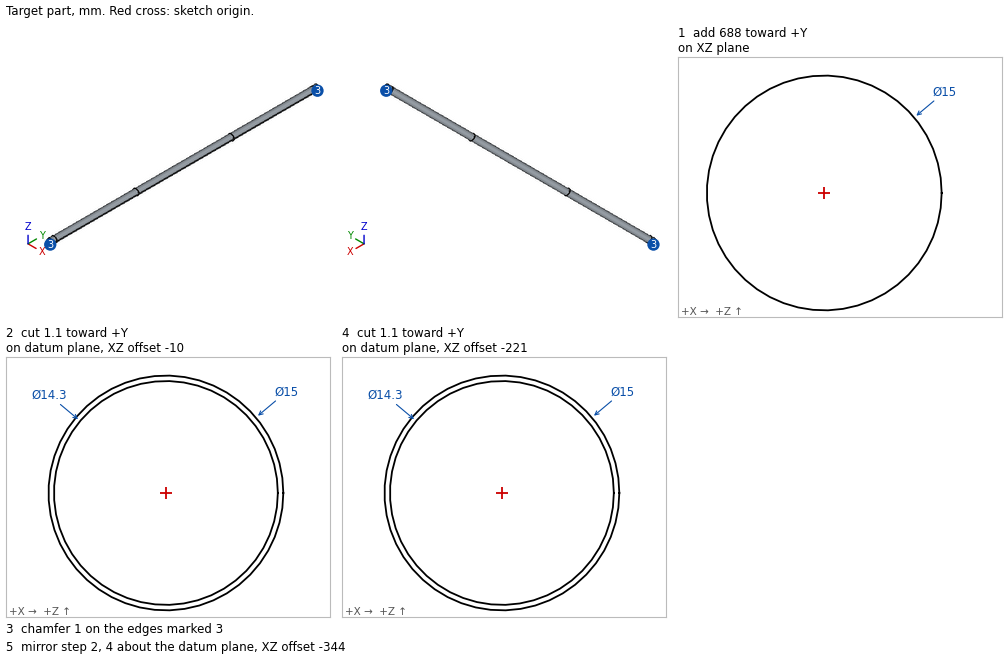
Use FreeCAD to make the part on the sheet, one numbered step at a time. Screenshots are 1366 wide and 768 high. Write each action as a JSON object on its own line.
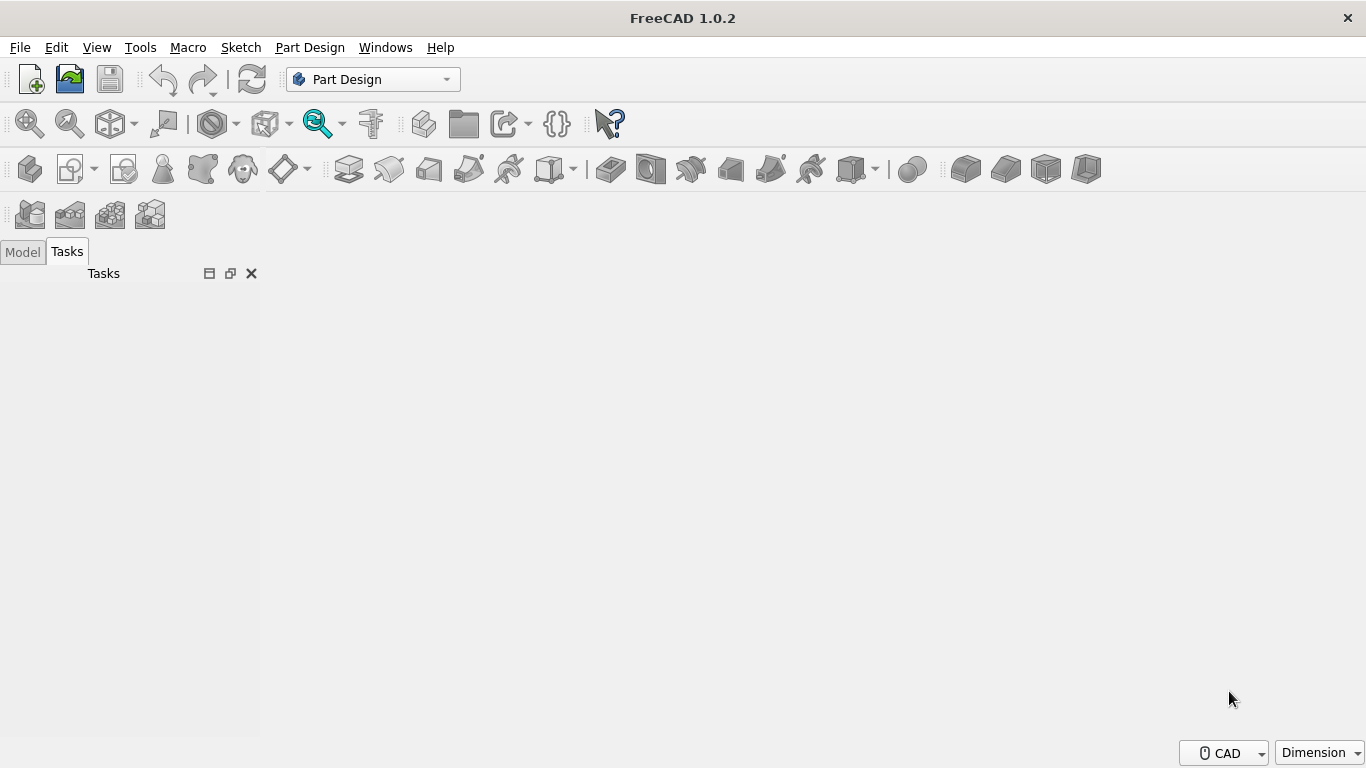
{"action": "left_click", "coordinate": [898, 80]}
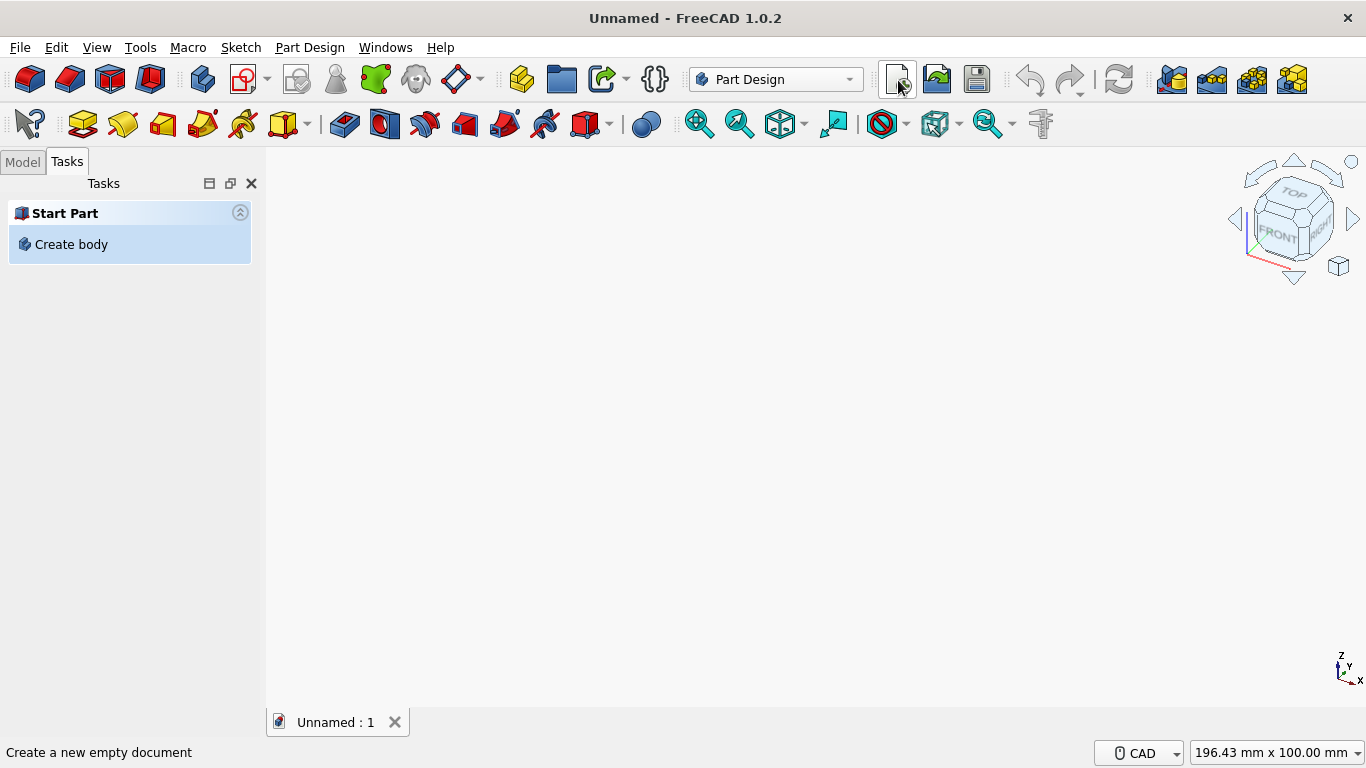
{"action": "left_click", "coordinate": [244, 80]}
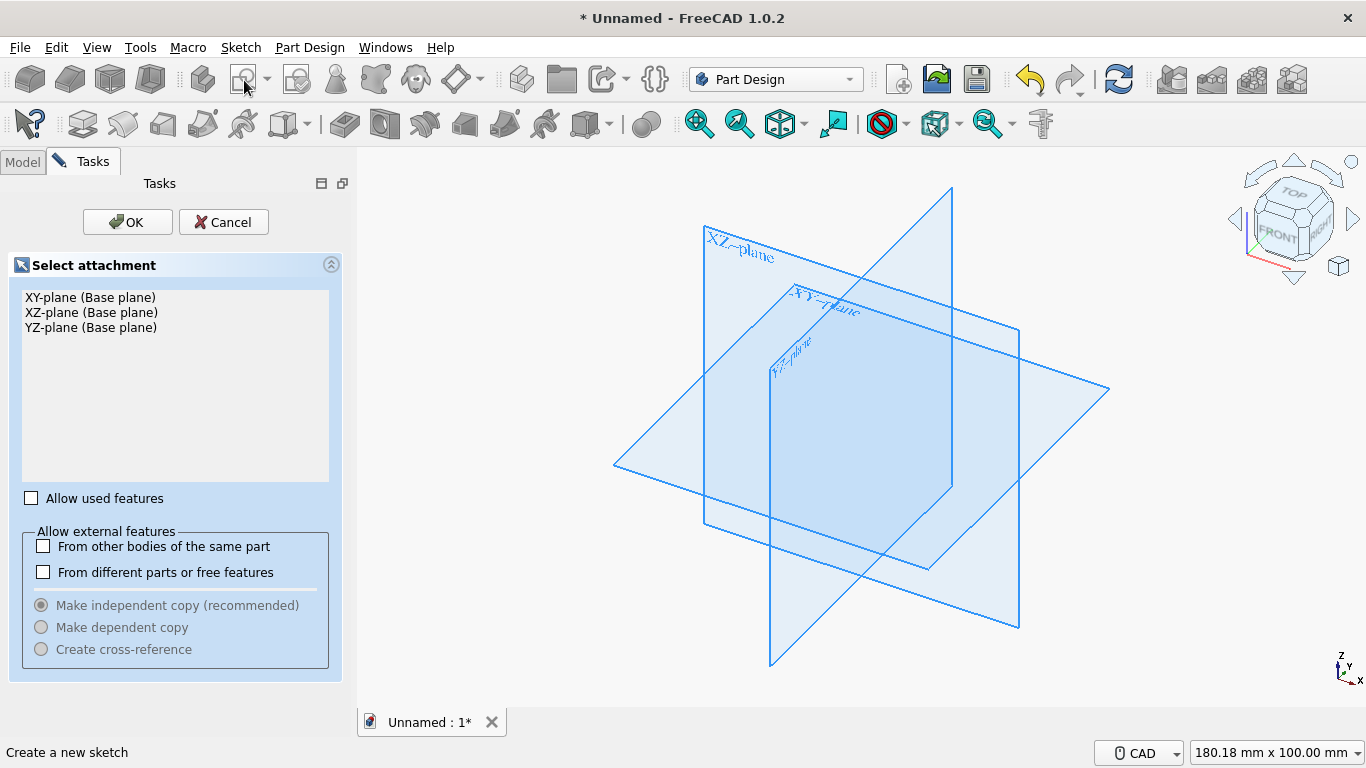
{"action": "left_click", "coordinate": [82, 312]}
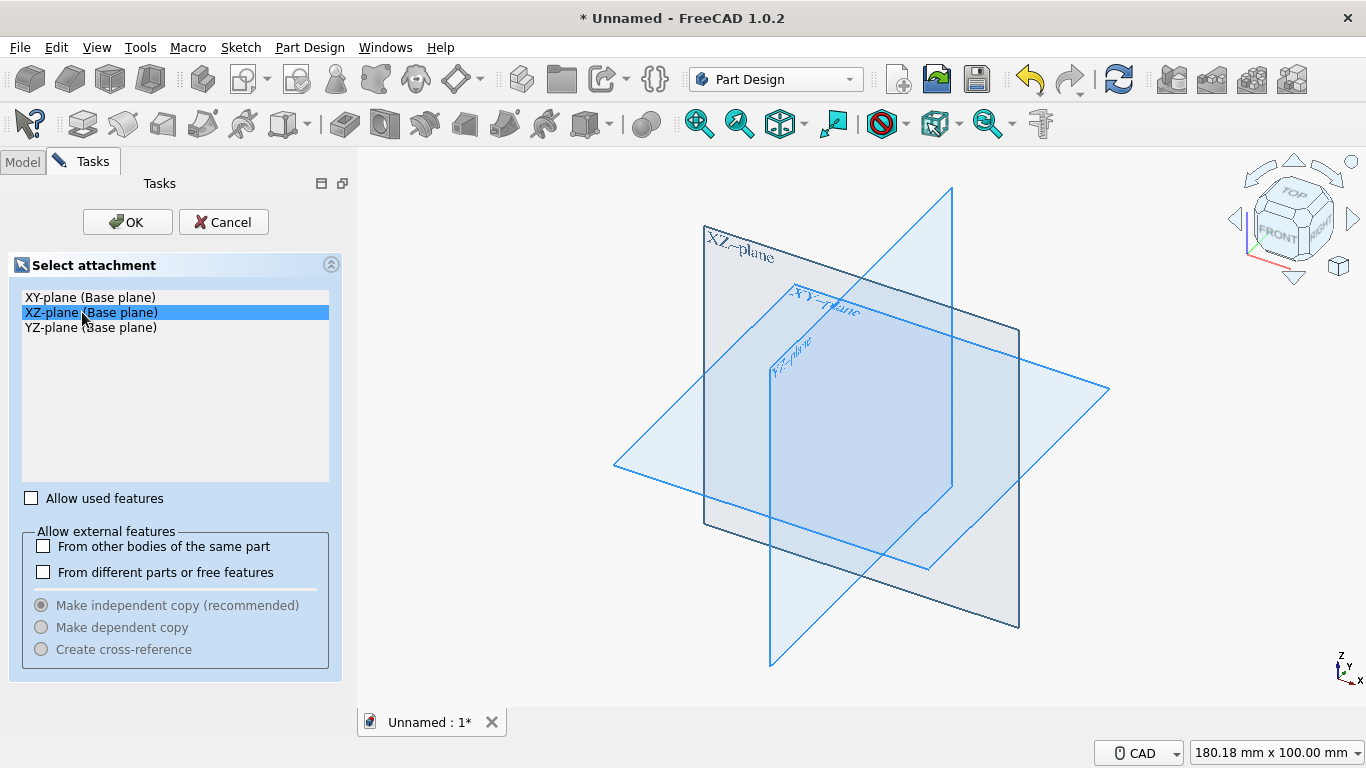
{"action": "left_click", "coordinate": [128, 222]}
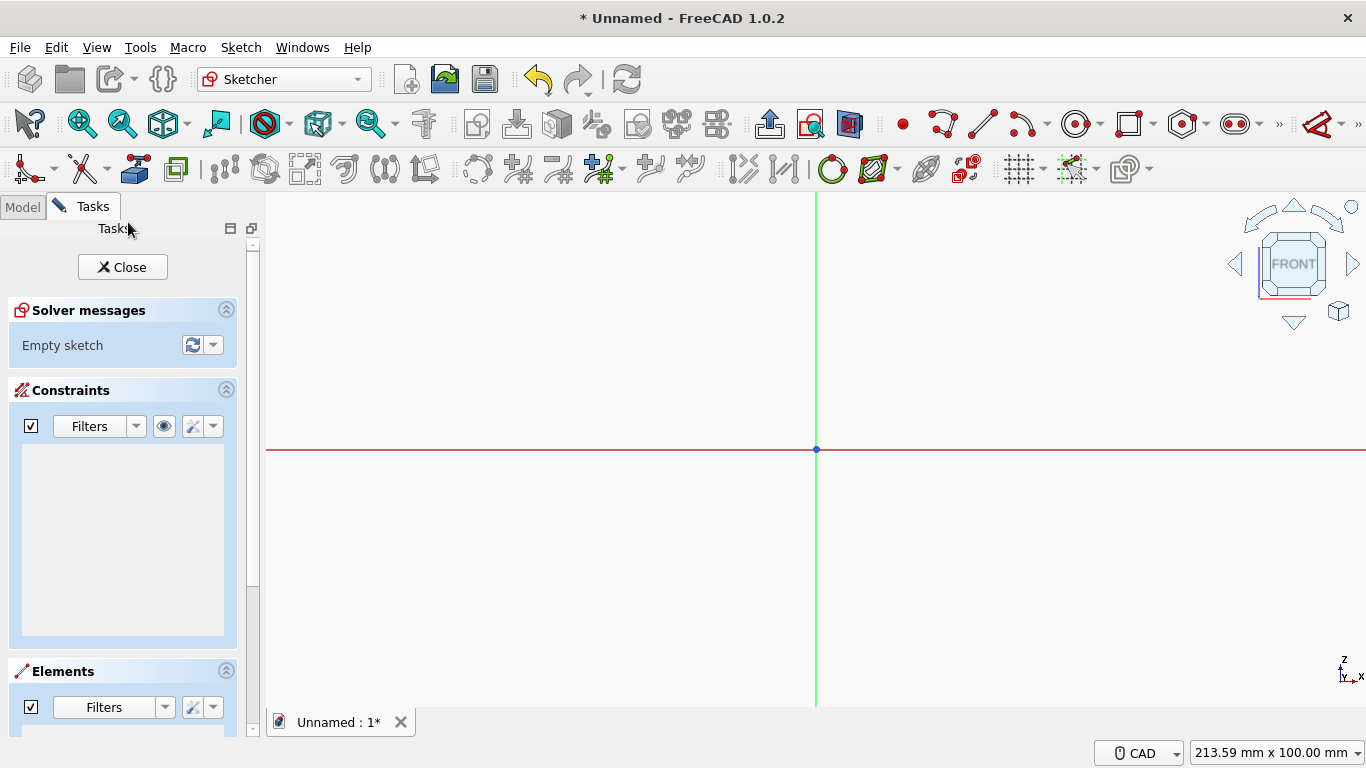
{"action": "scroll", "coordinate": [838, 449], "scroll_direction": "up", "scroll_amount": 7}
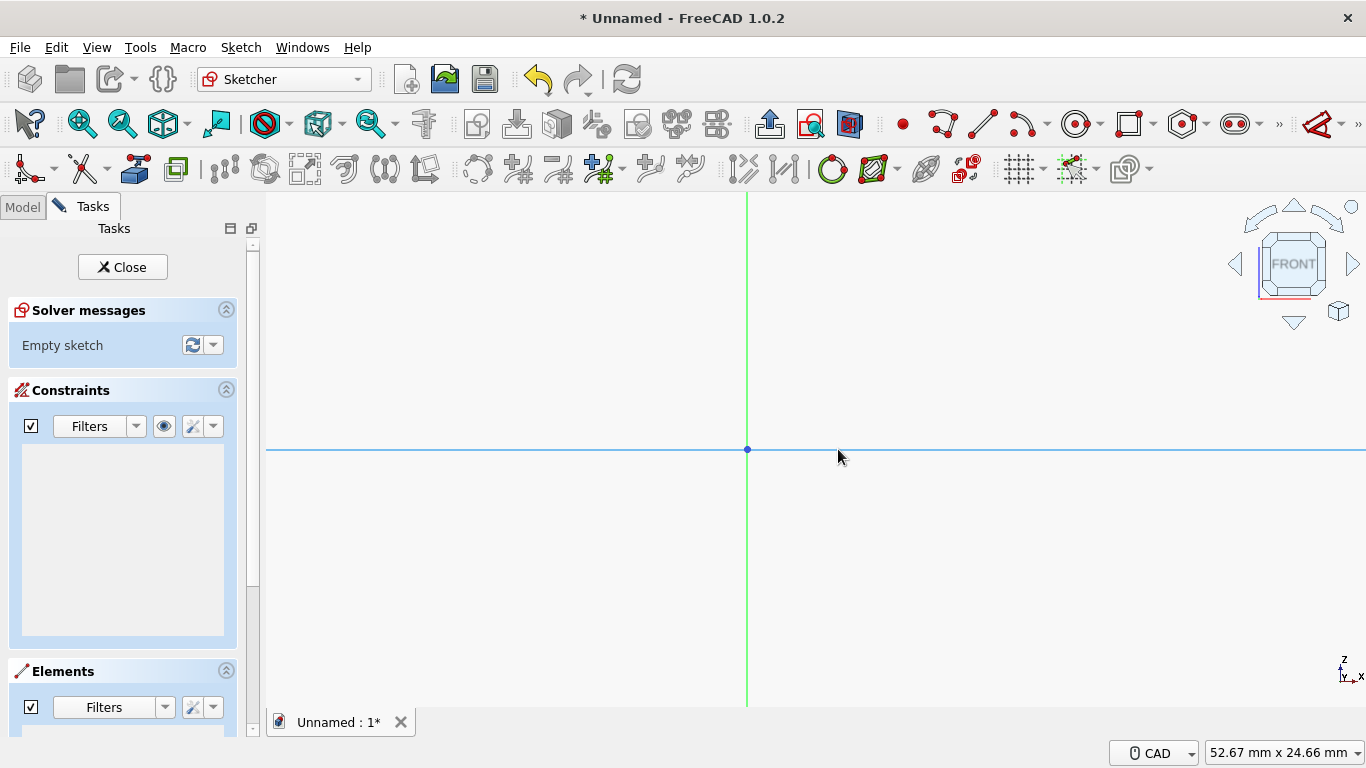
{"action": "left_click", "coordinate": [1076, 124]}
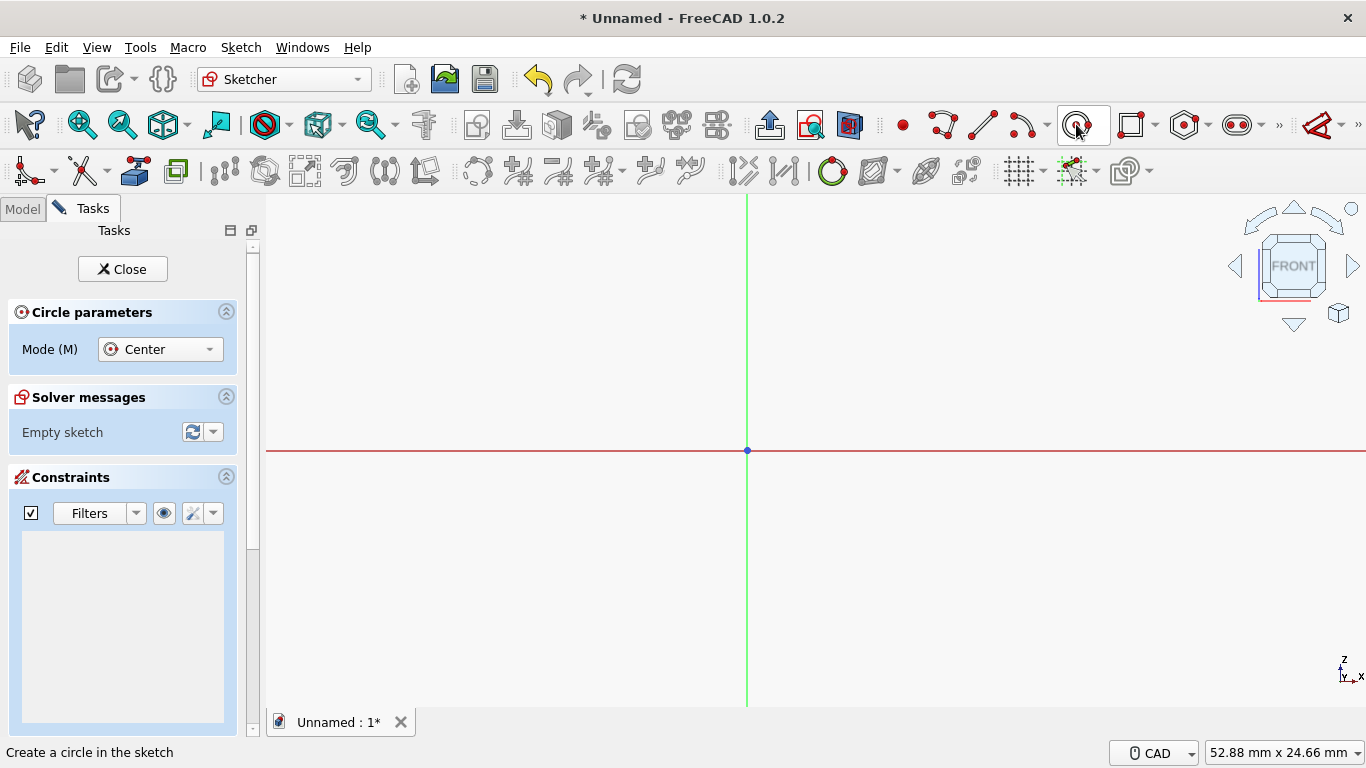
{"action": "left_click", "coordinate": [747, 450]}
{"action": "mouse_move", "coordinate": [858, 340]}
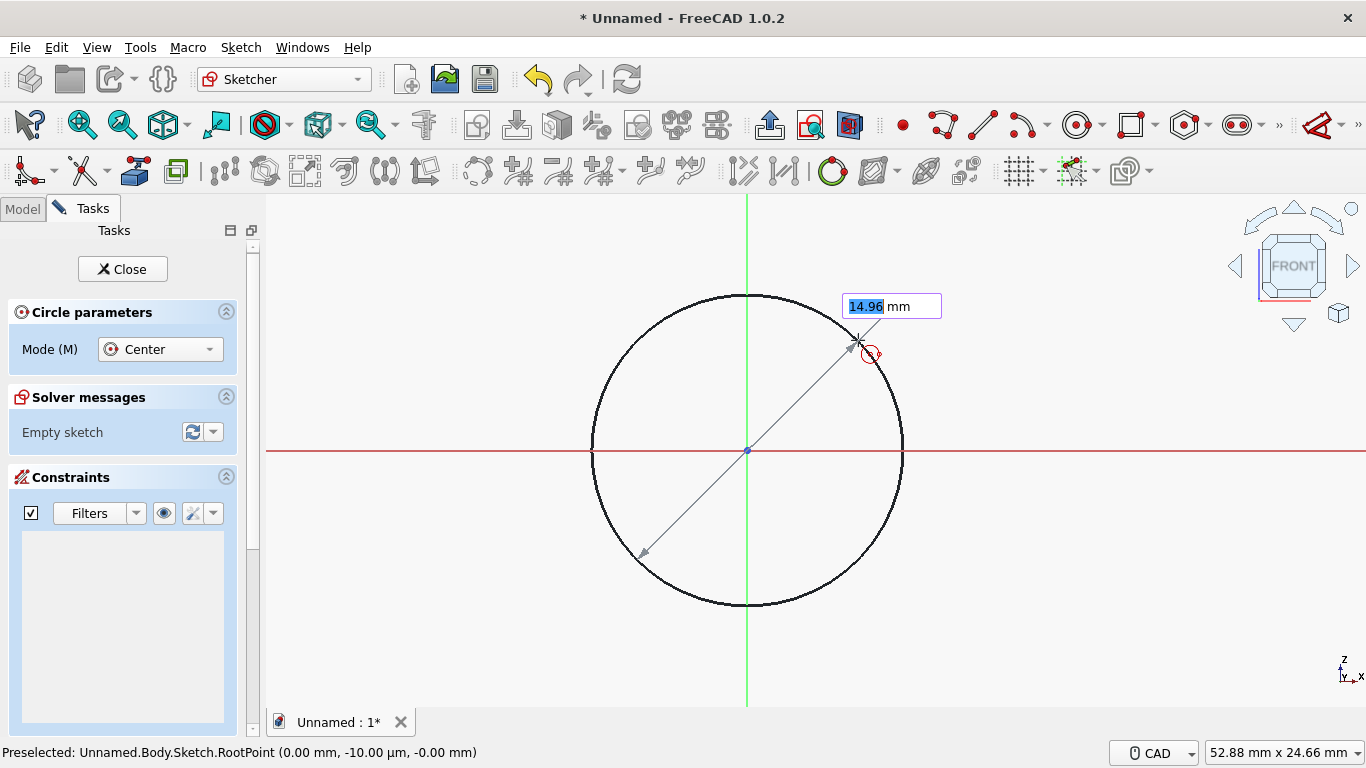
{"action": "type", "text": "15"}
{"action": "key", "text": "Return"}
{"action": "key", "text": "Escape"}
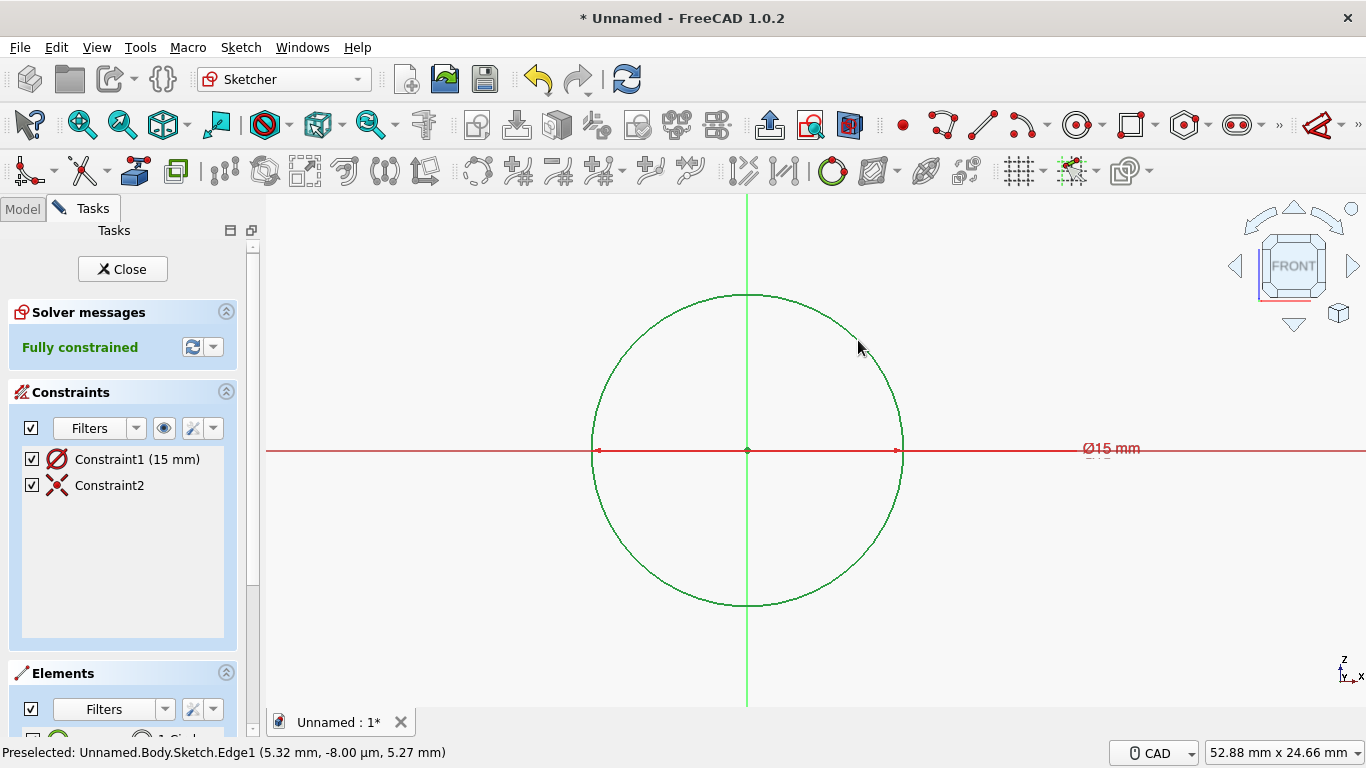
{"action": "left_click", "coordinate": [123, 269]}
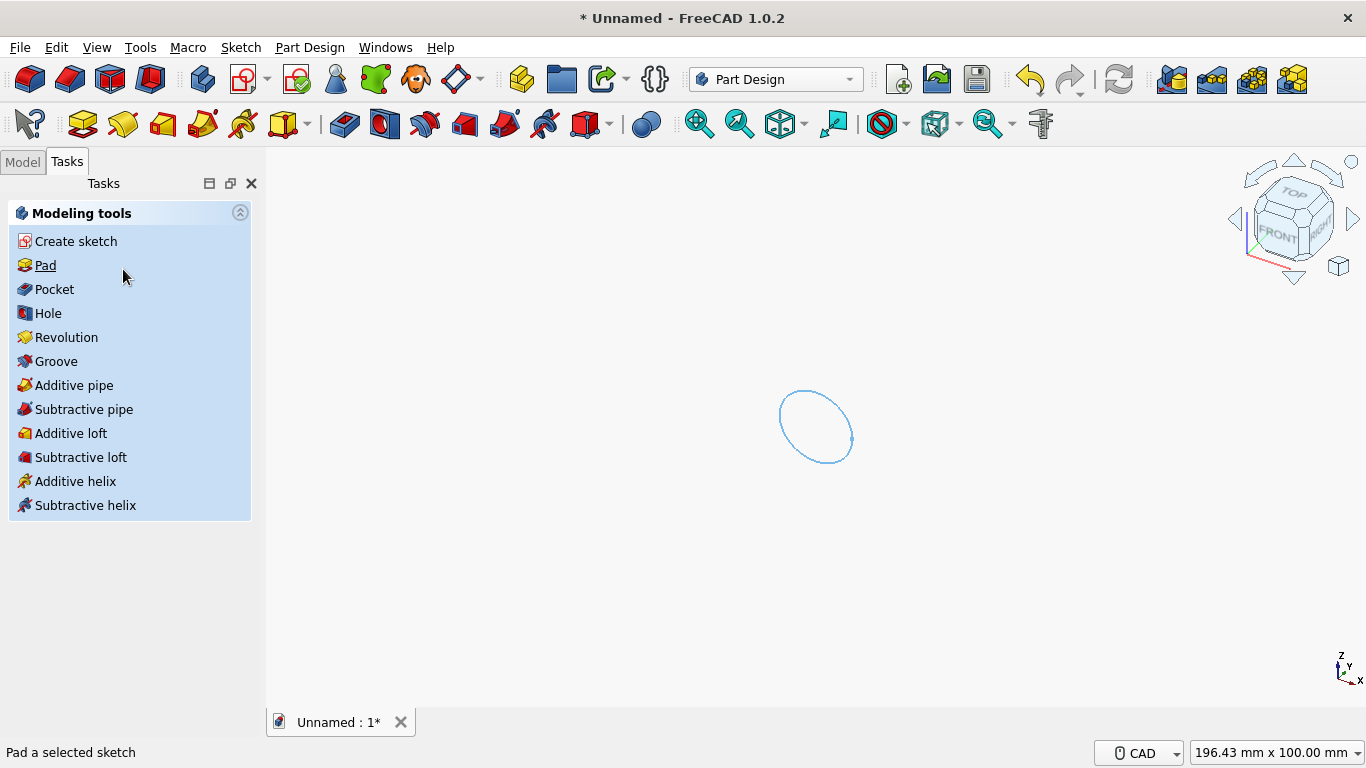
{"action": "left_click", "coordinate": [84, 124]}